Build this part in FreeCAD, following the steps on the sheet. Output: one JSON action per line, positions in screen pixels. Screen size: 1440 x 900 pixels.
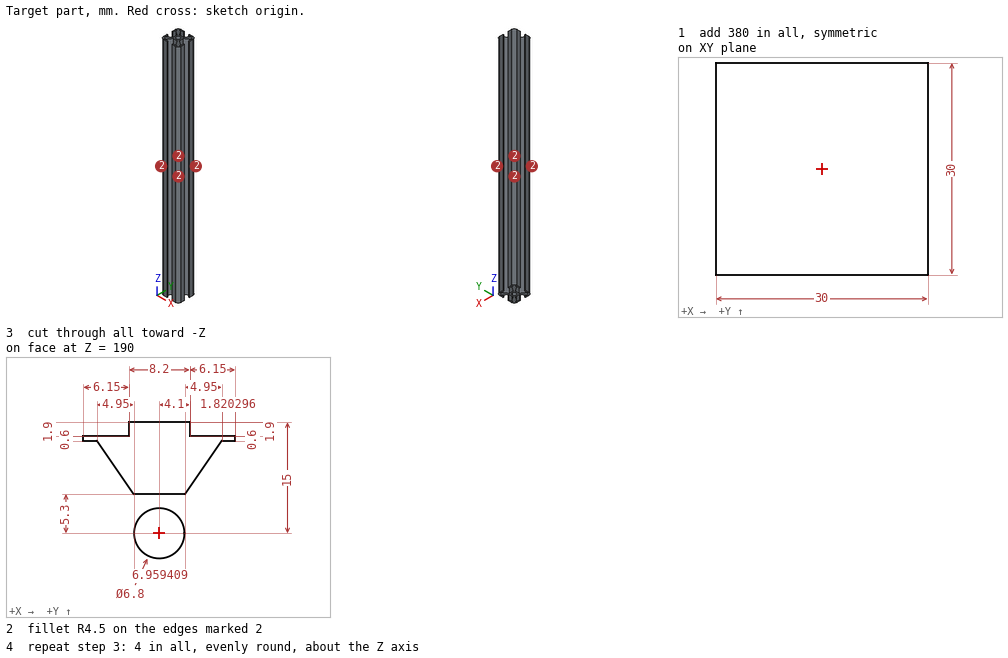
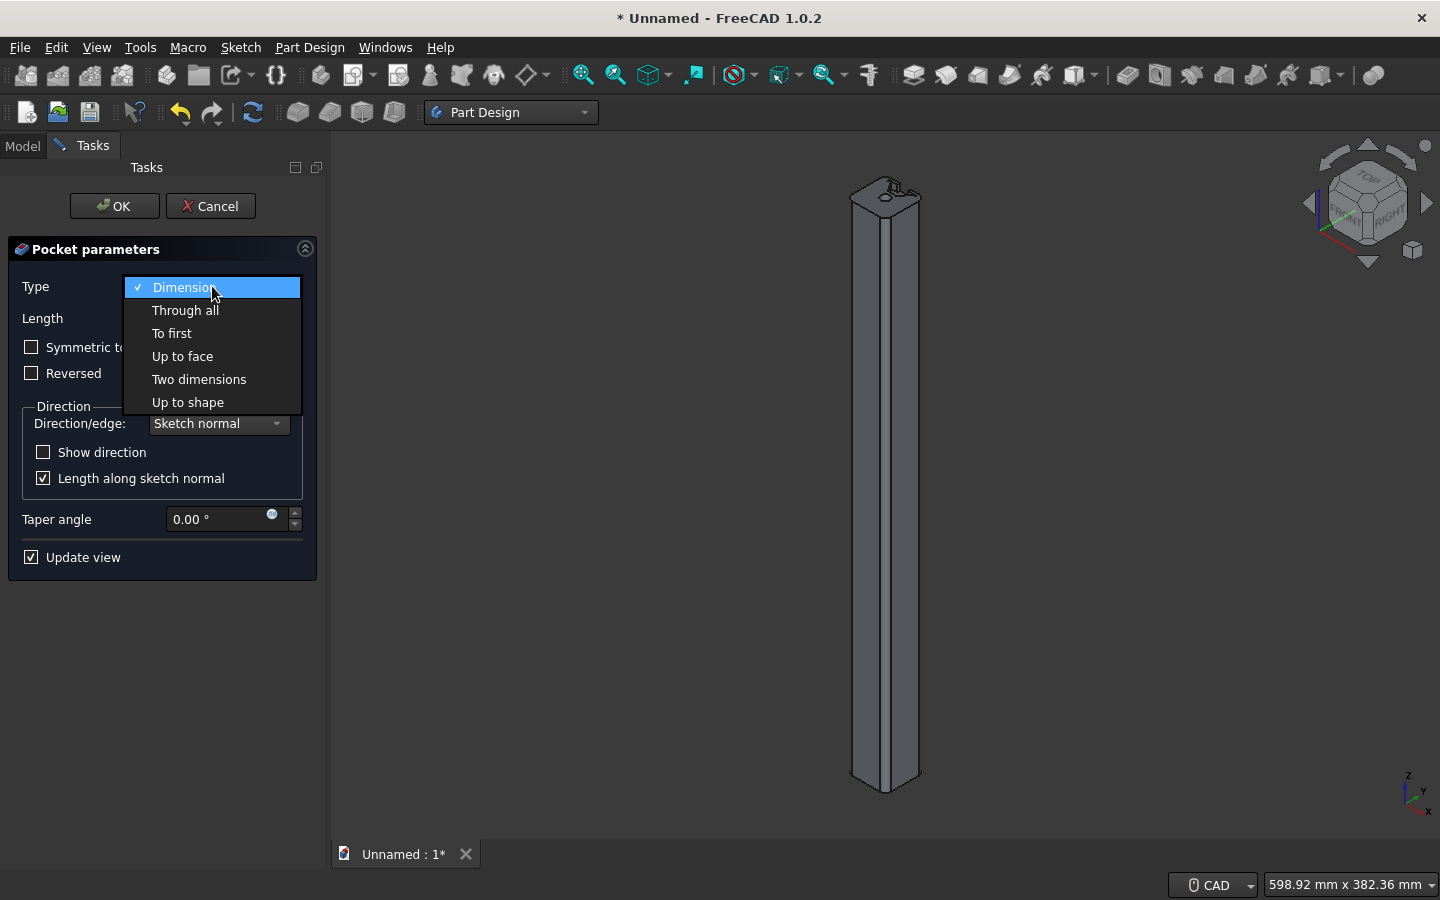
{"action": "left_click", "coordinate": [212, 310]}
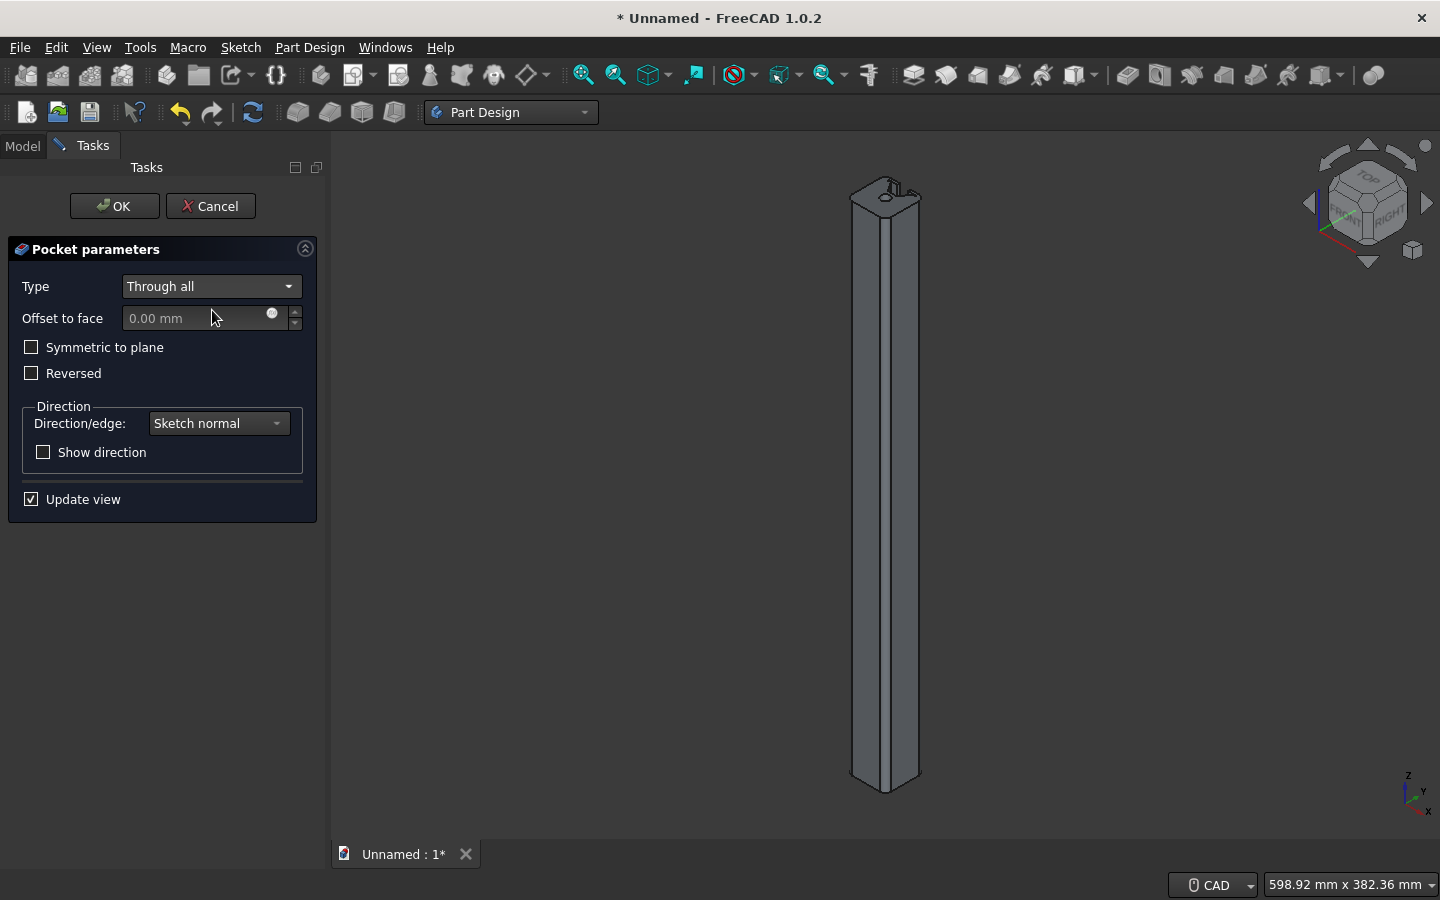
{"action": "left_click", "coordinate": [115, 206]}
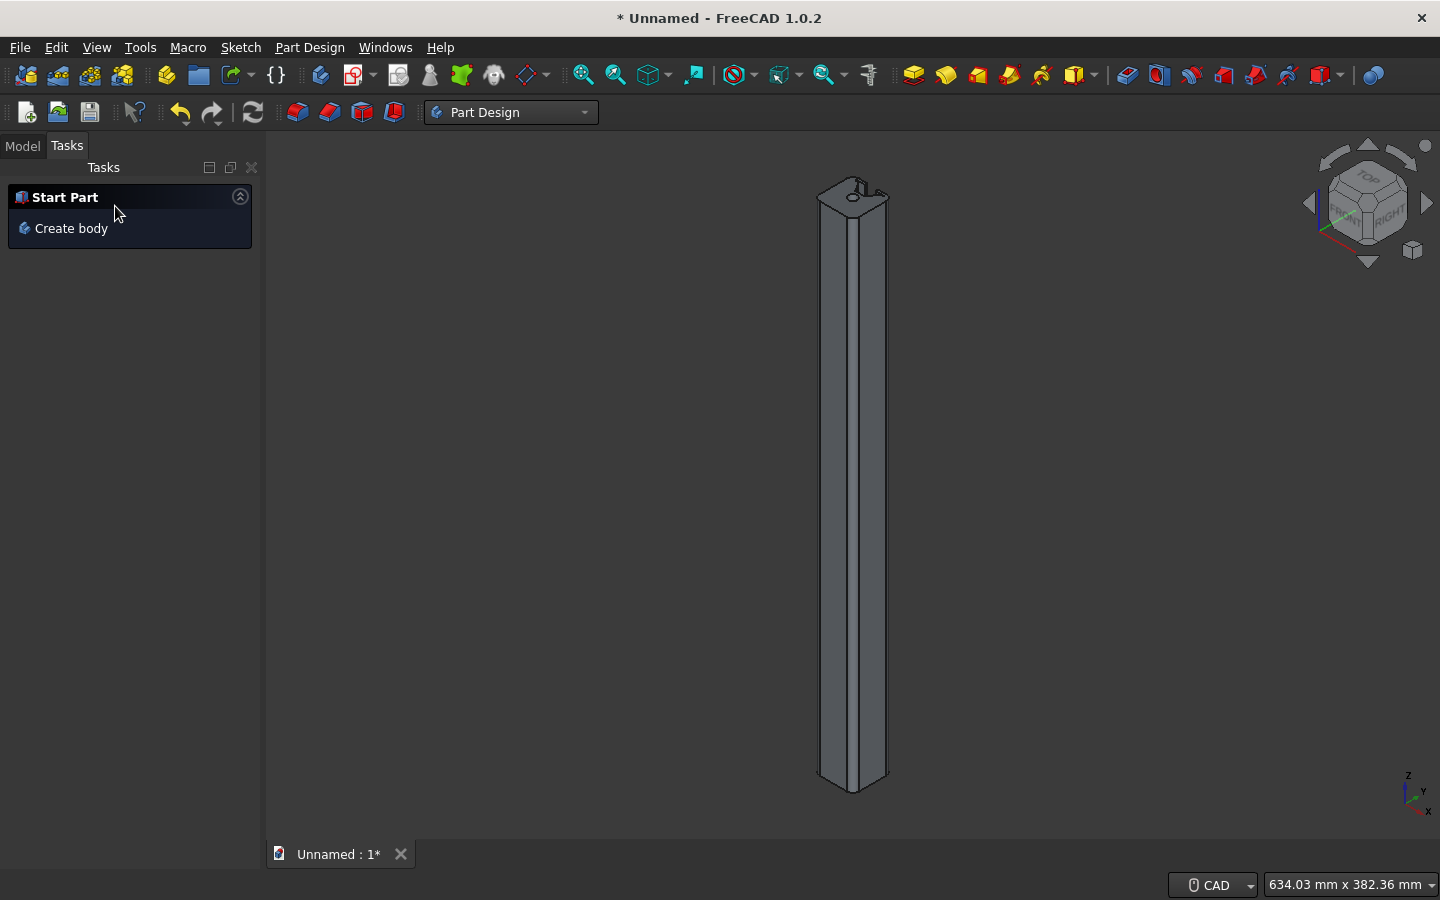
{"action": "left_click", "coordinate": [23, 145]}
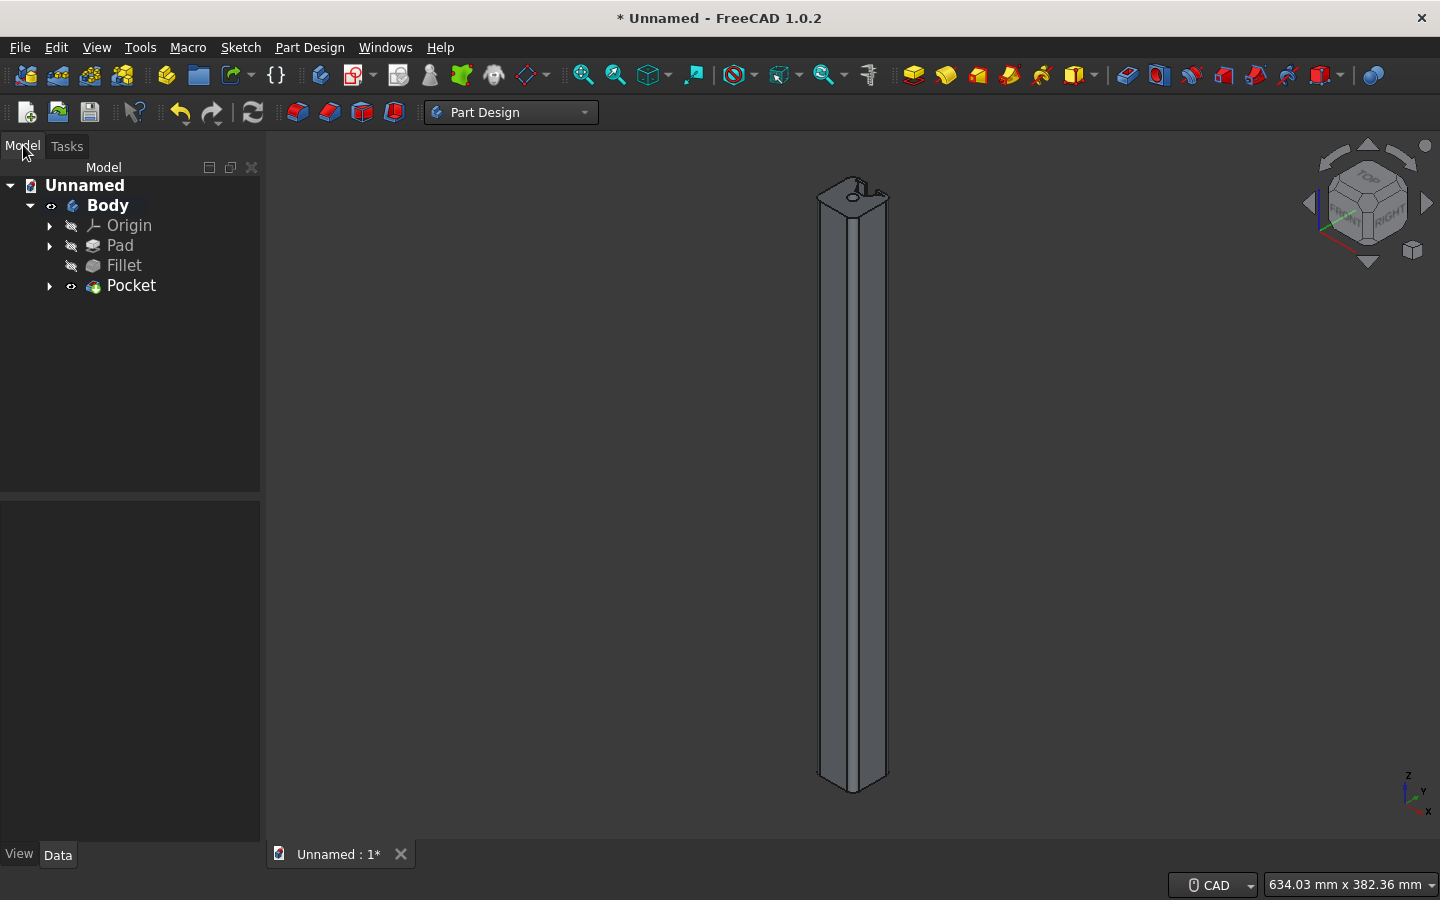
{"action": "left_click", "coordinate": [116, 286]}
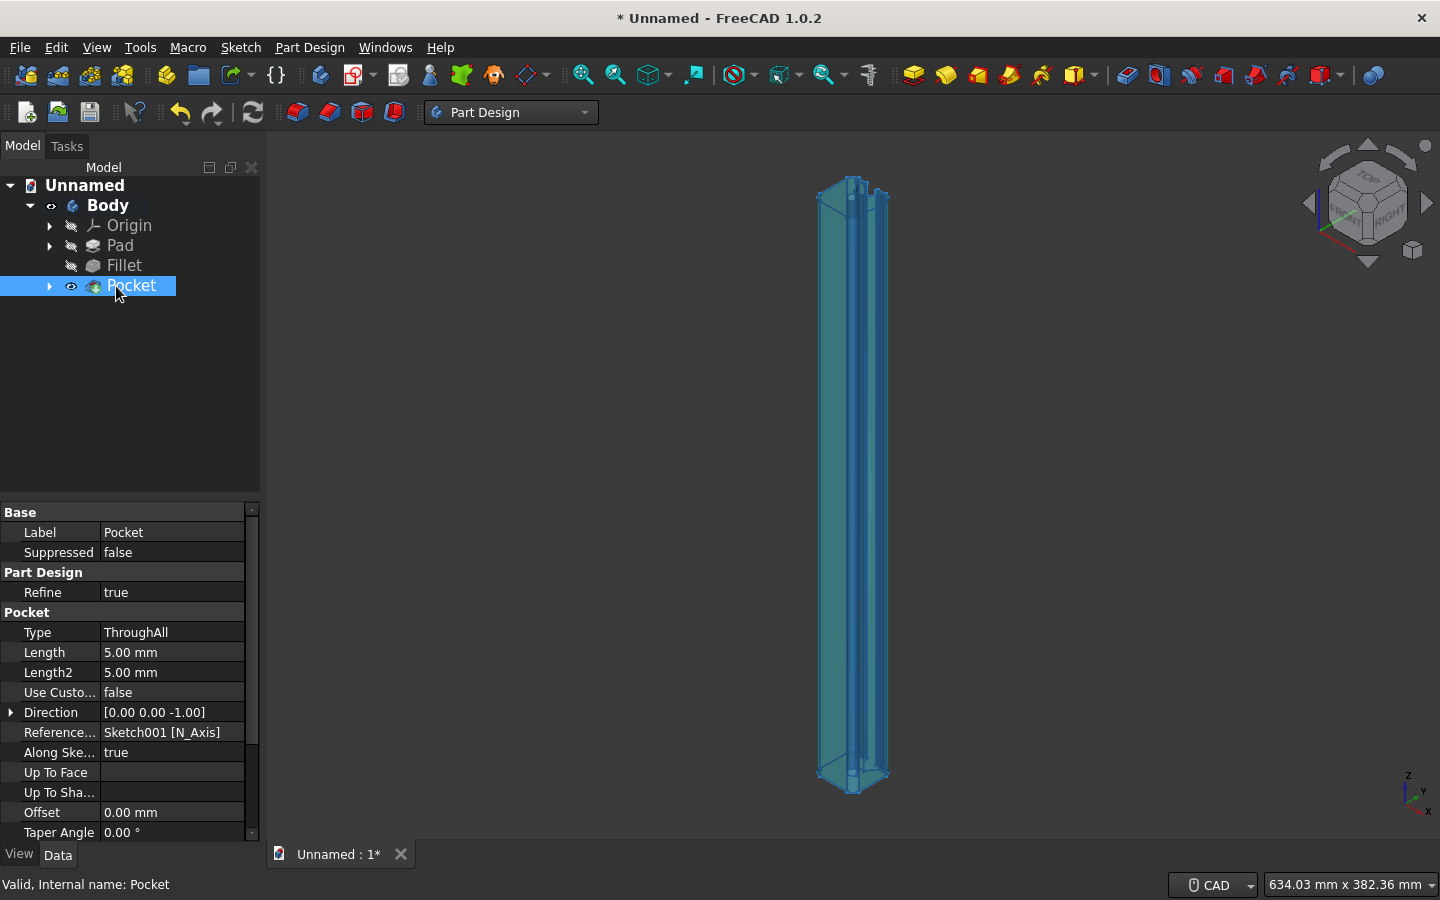
{"action": "left_click", "coordinate": [90, 76]}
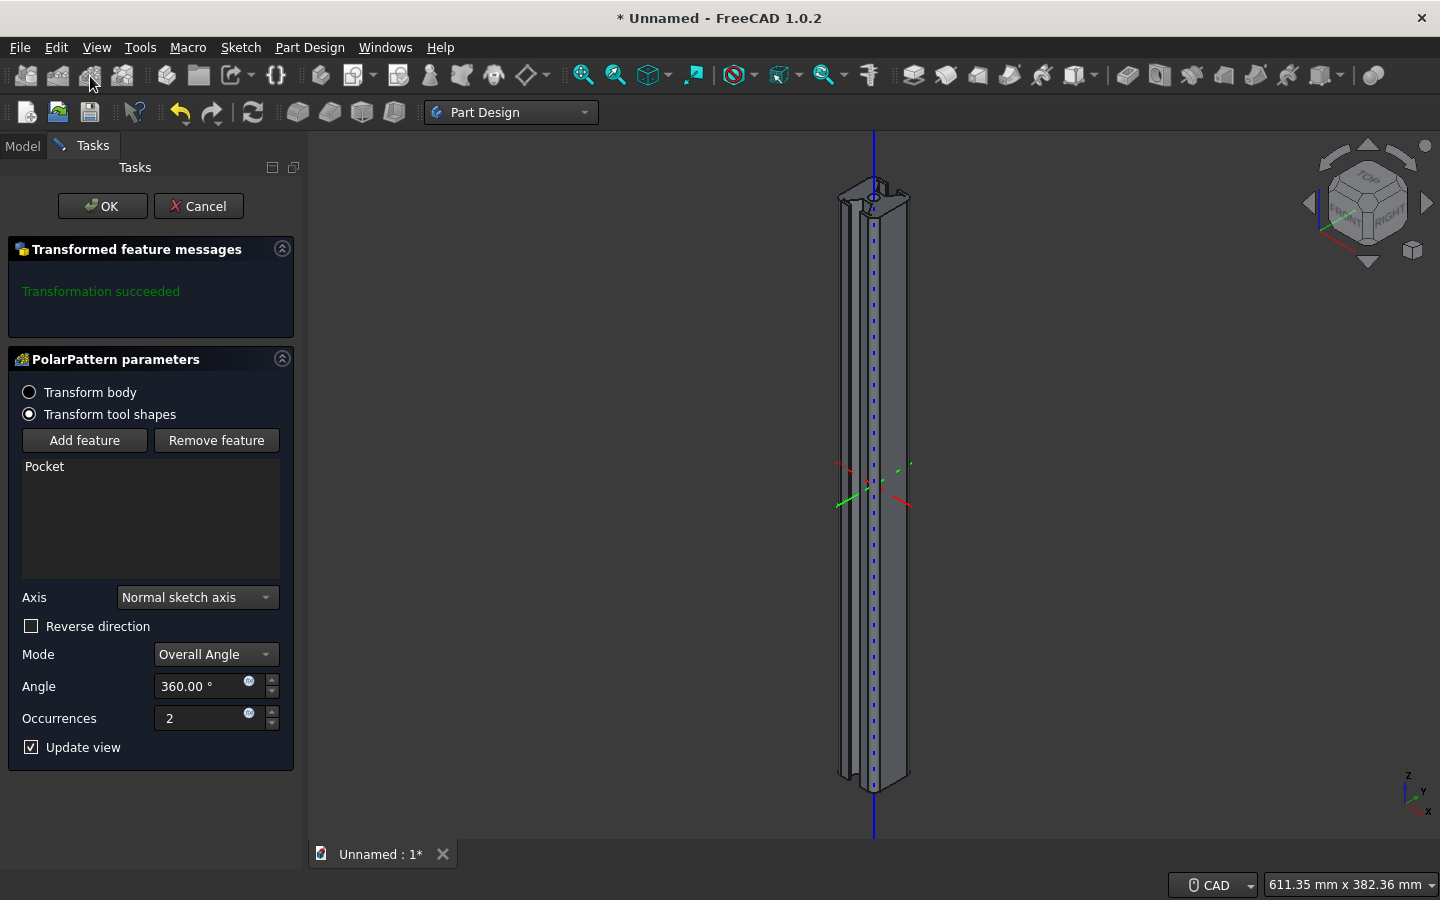
{"action": "left_click", "coordinate": [198, 598]}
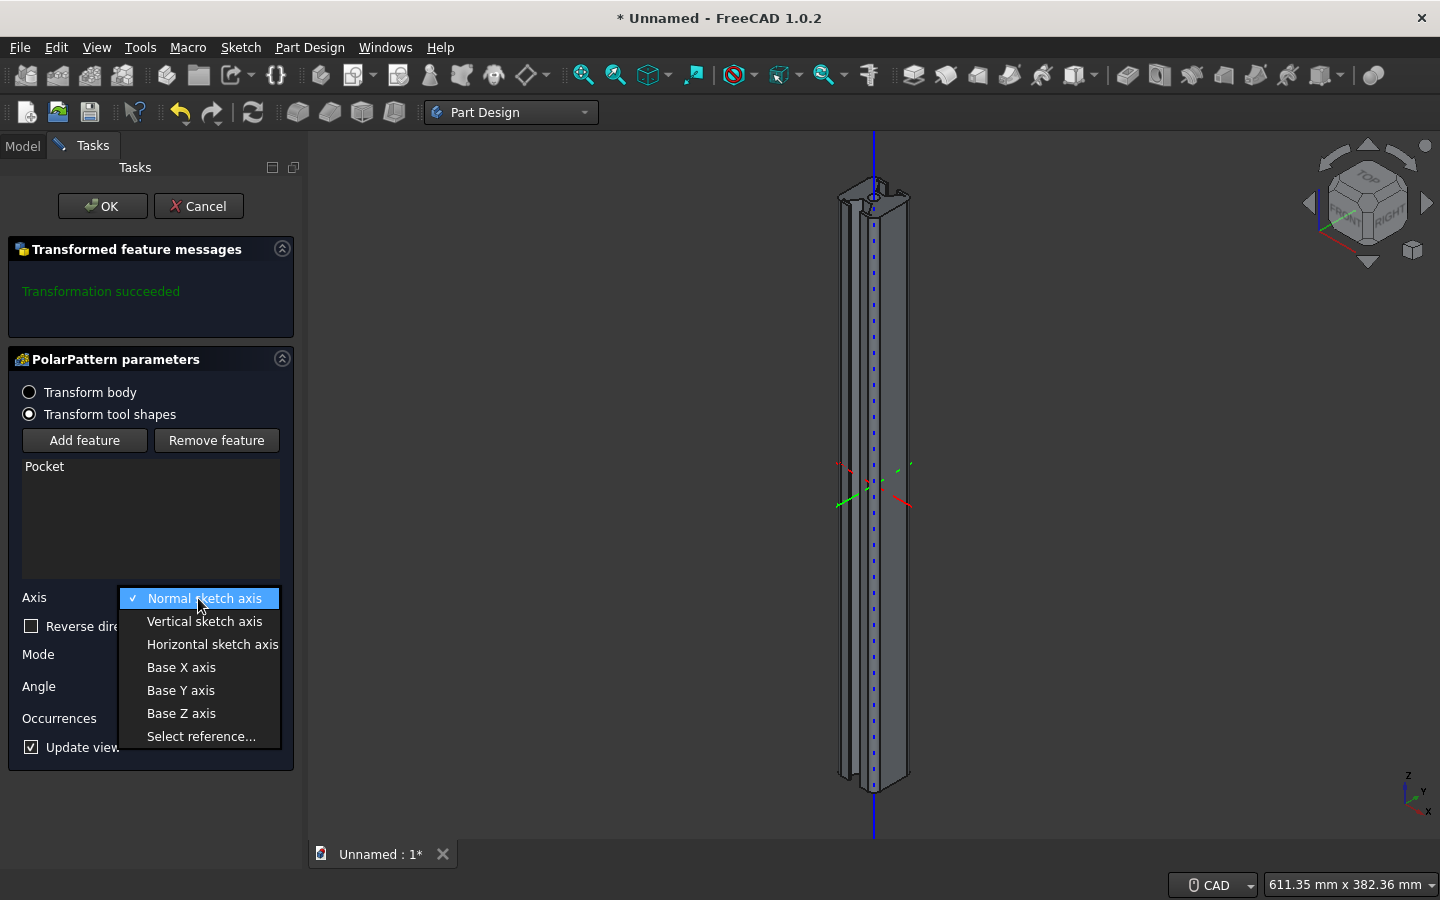
{"action": "left_click", "coordinate": [198, 714]}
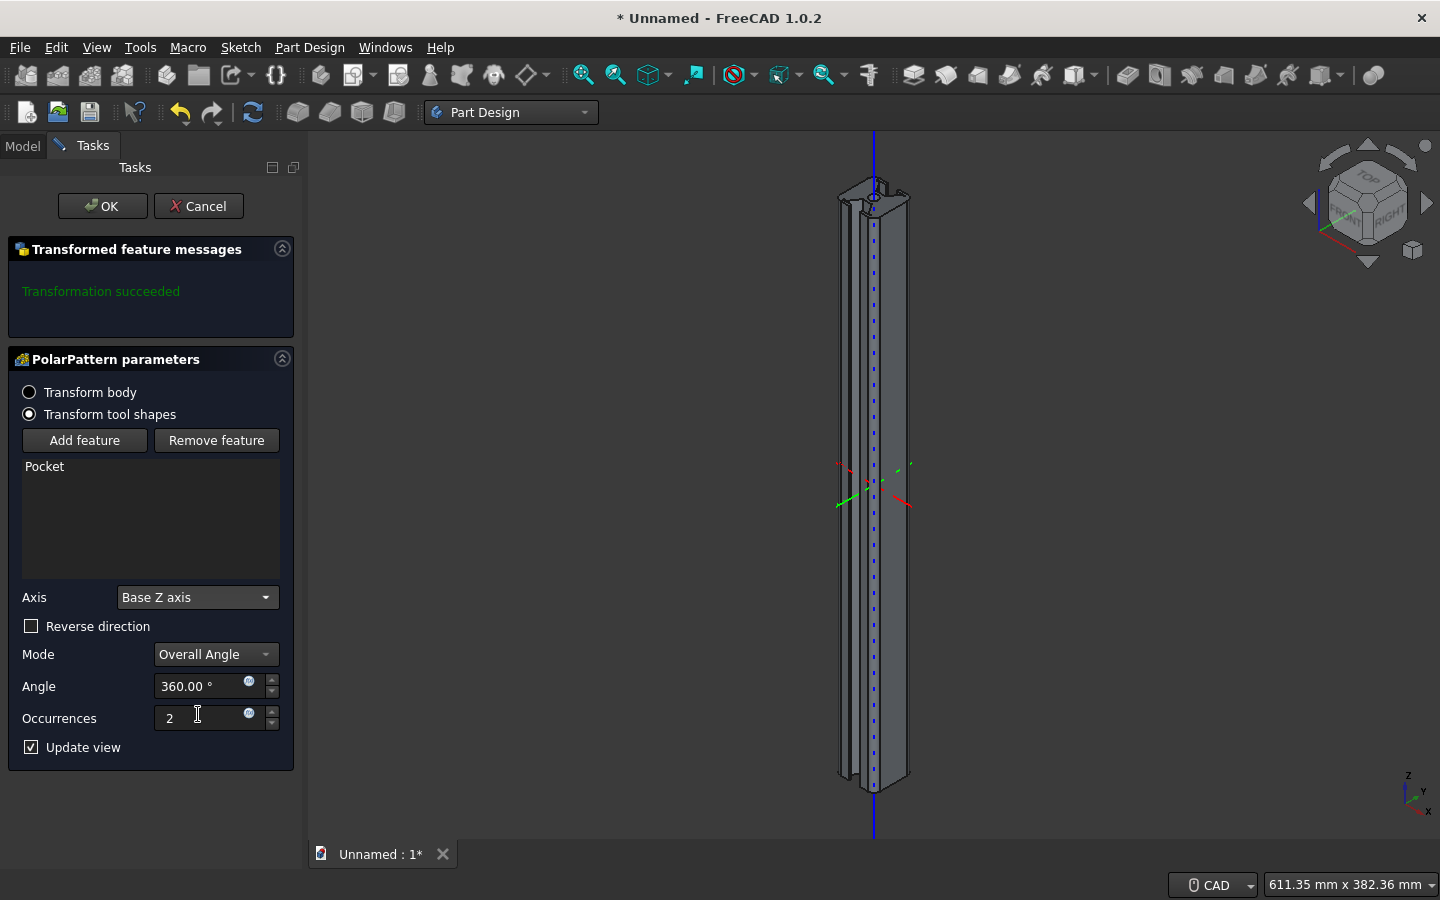
{"action": "triple_click", "coordinate": [209, 718]}